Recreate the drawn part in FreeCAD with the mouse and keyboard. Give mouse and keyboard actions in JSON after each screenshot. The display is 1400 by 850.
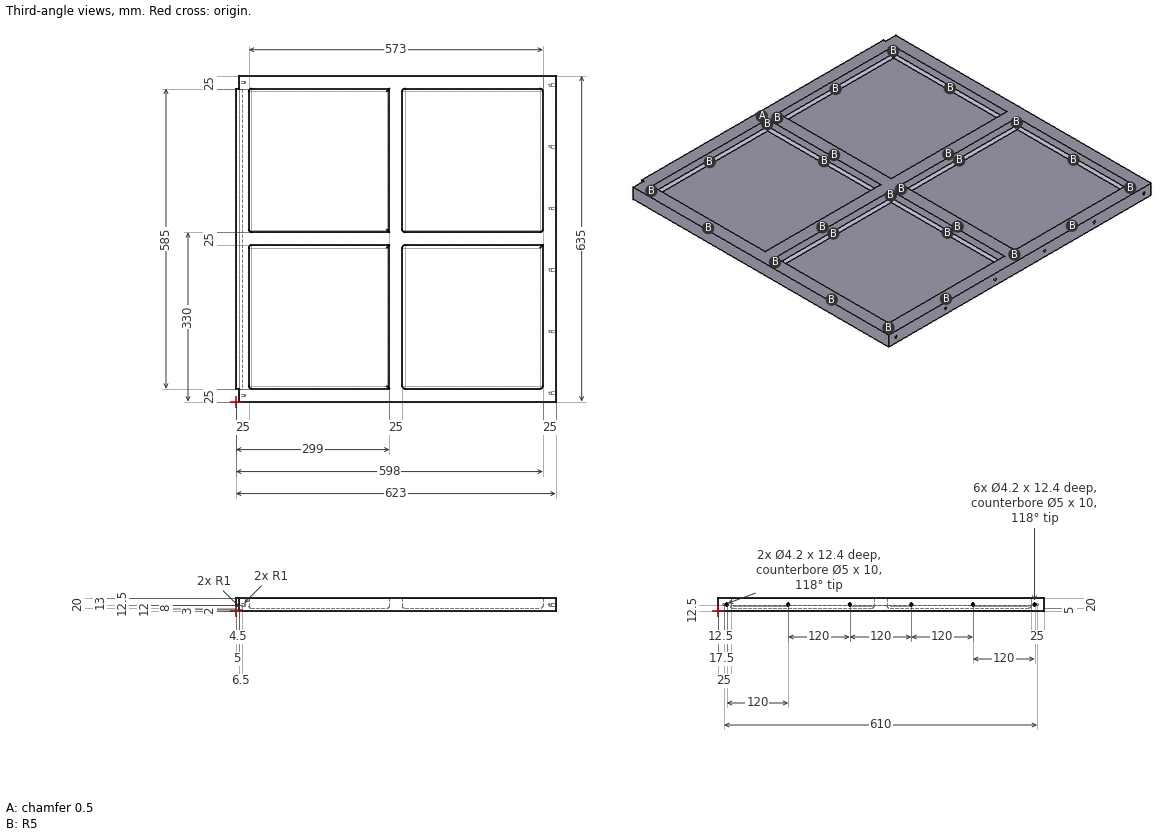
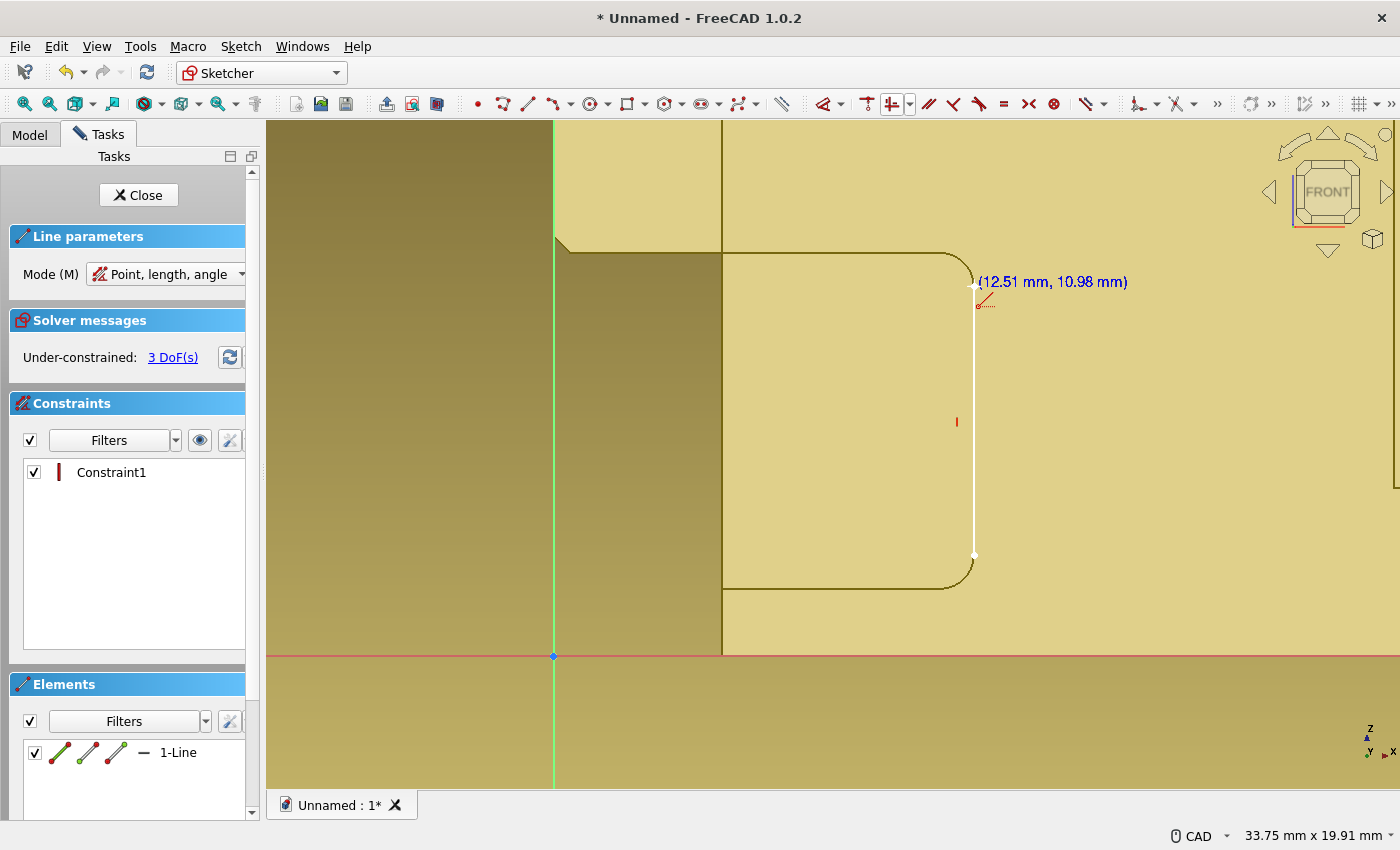
{"action": "key", "text": "g m"}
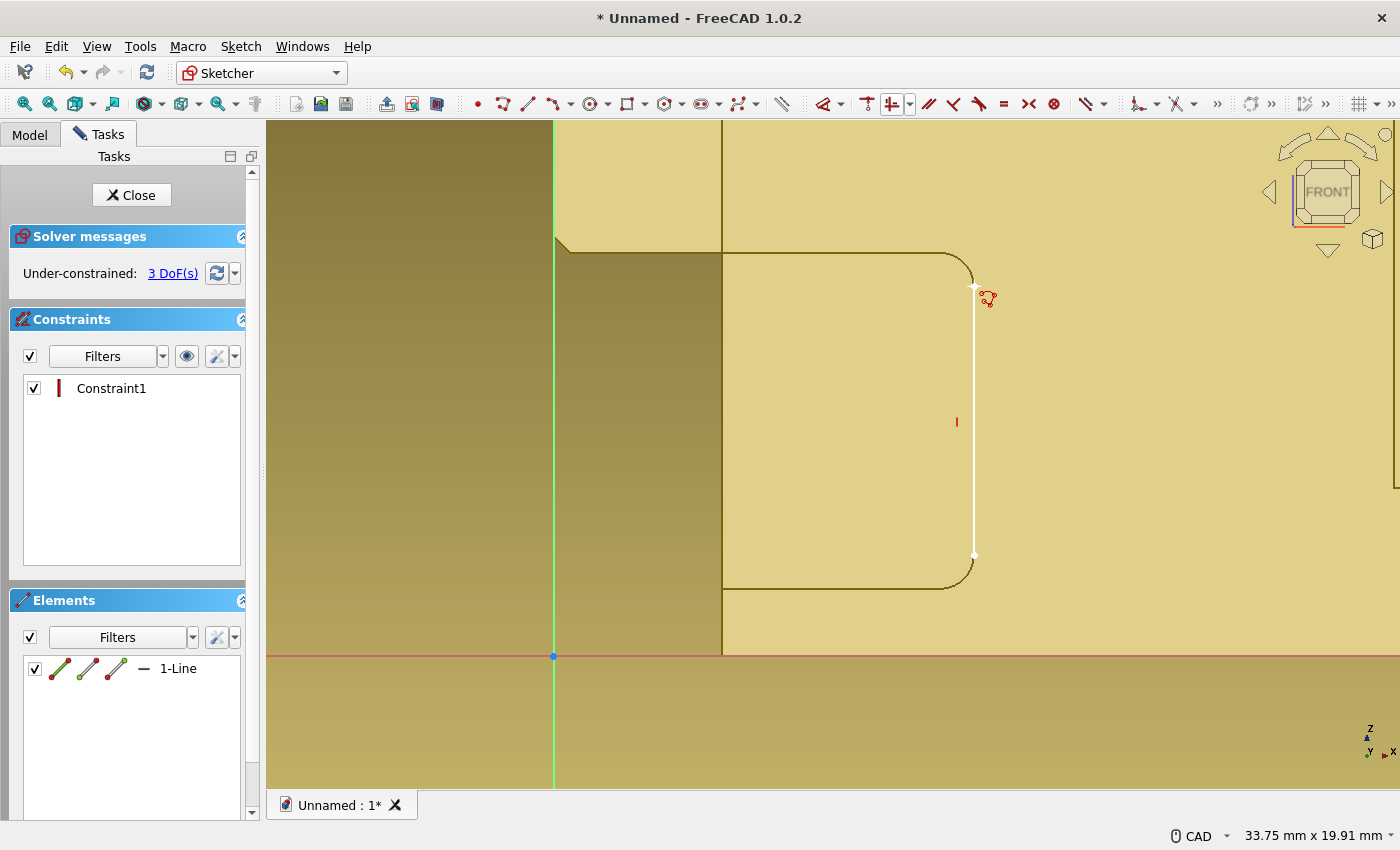
{"action": "left_click", "coordinate": [940, 253]}
{"action": "left_click", "coordinate": [722, 253]}
{"action": "left_click", "coordinate": [722, 589]}
{"action": "left_click", "coordinate": [940, 589]}
{"action": "right_click", "coordinate": [940, 589]}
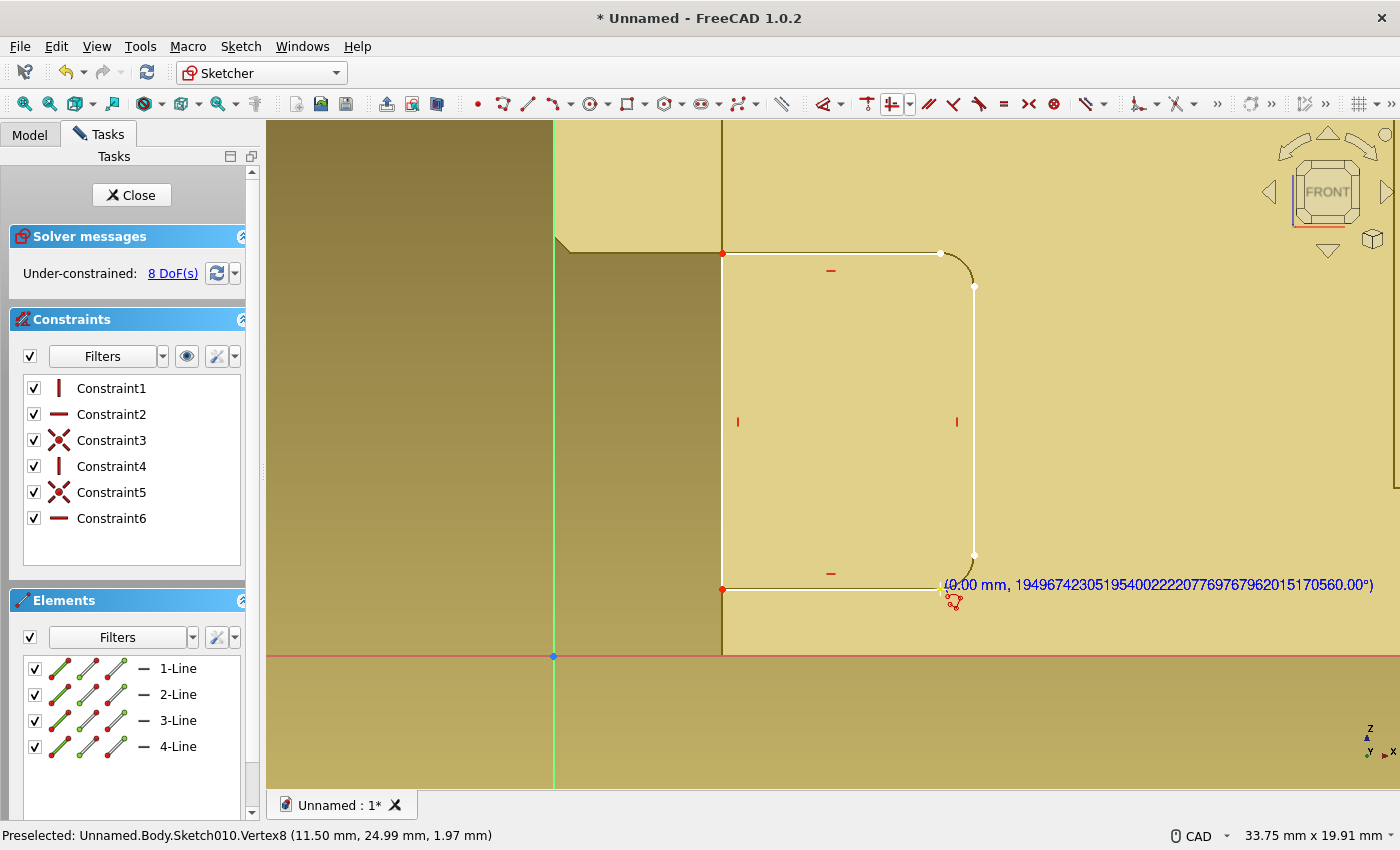
{"action": "key", "text": "g 3 a"}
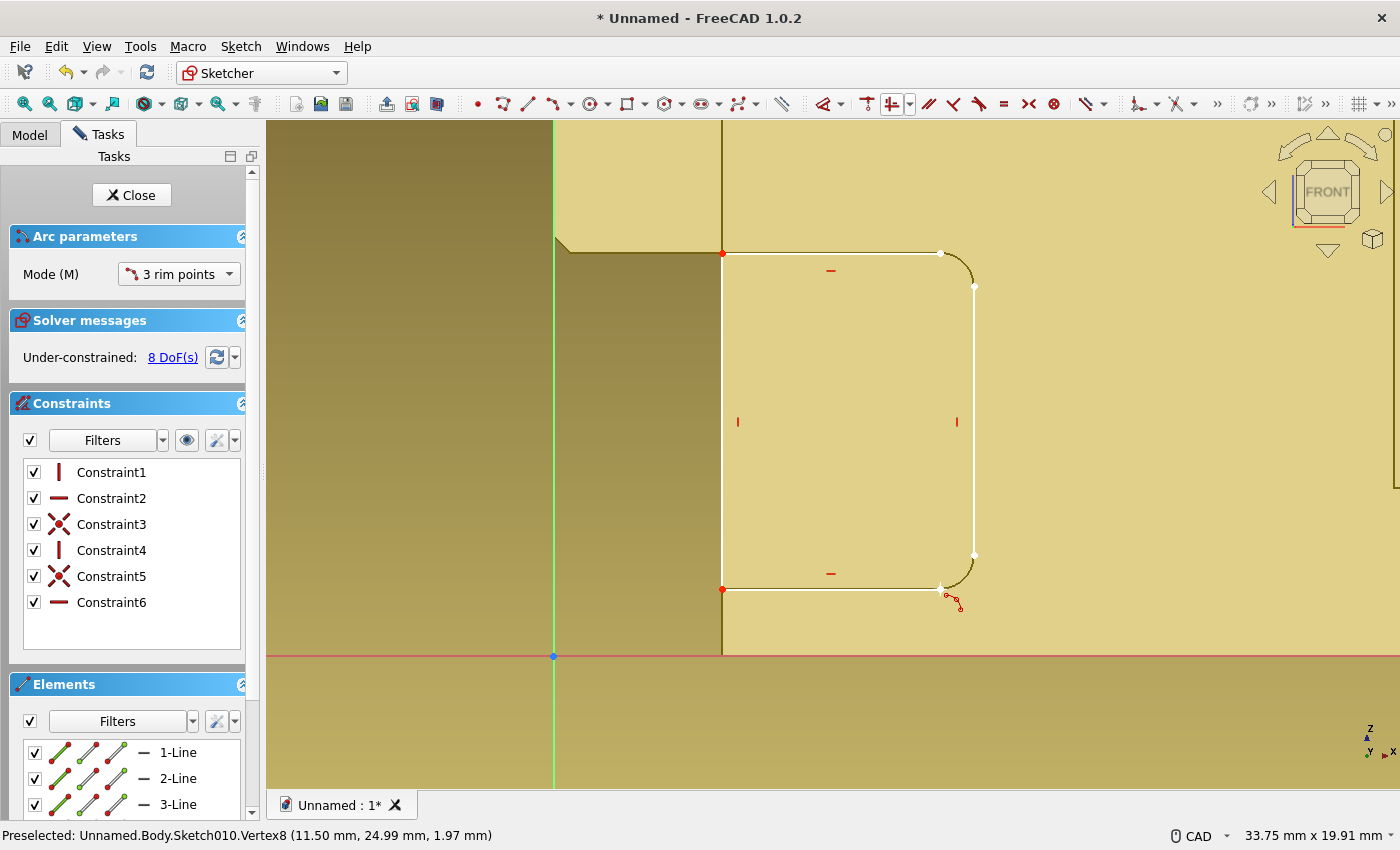
{"action": "left_click", "coordinate": [974, 287]}
{"action": "left_click", "coordinate": [940, 254]}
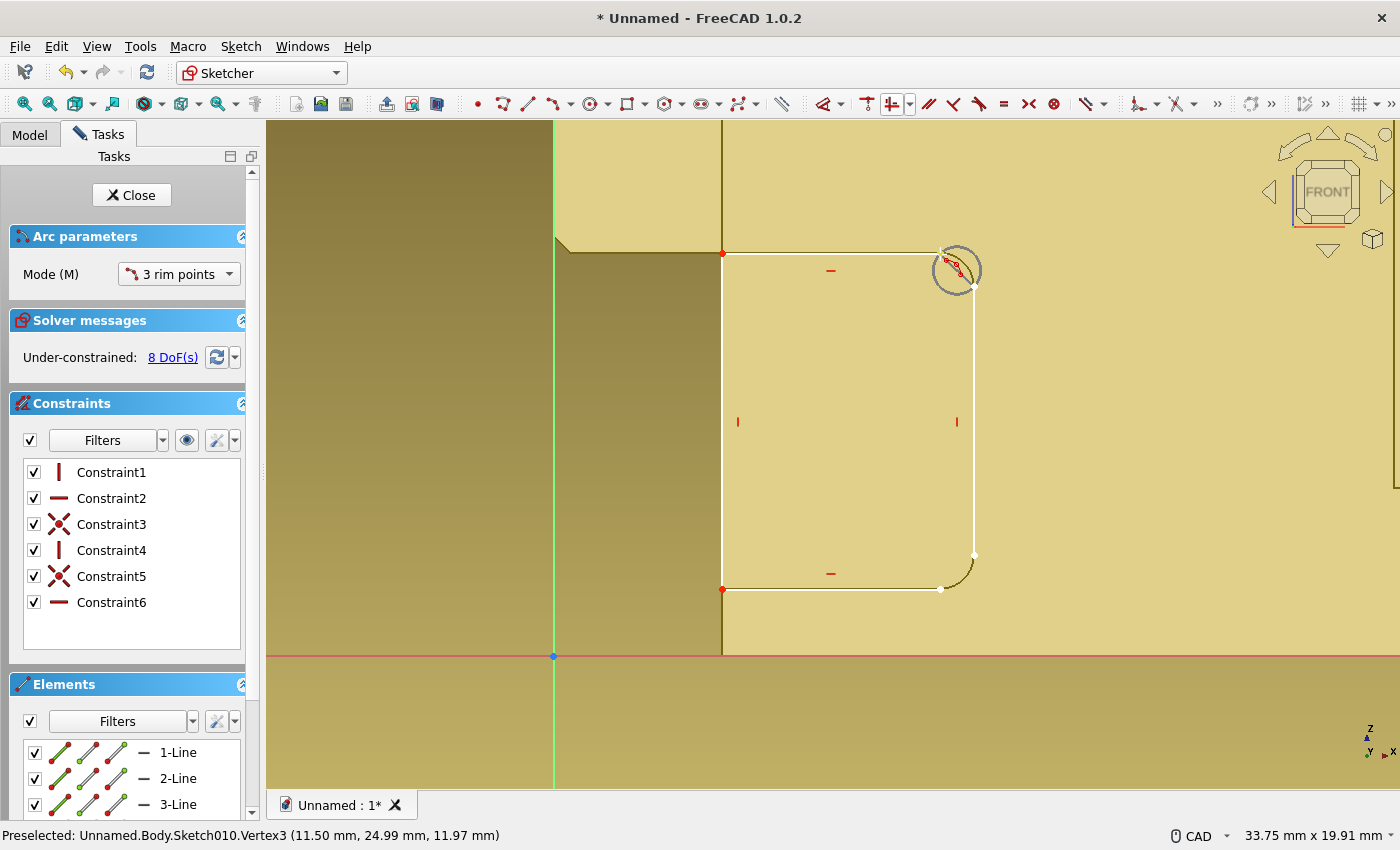
{"action": "scroll", "coordinate": [964, 263], "scroll_direction": "up", "scroll_amount": 3}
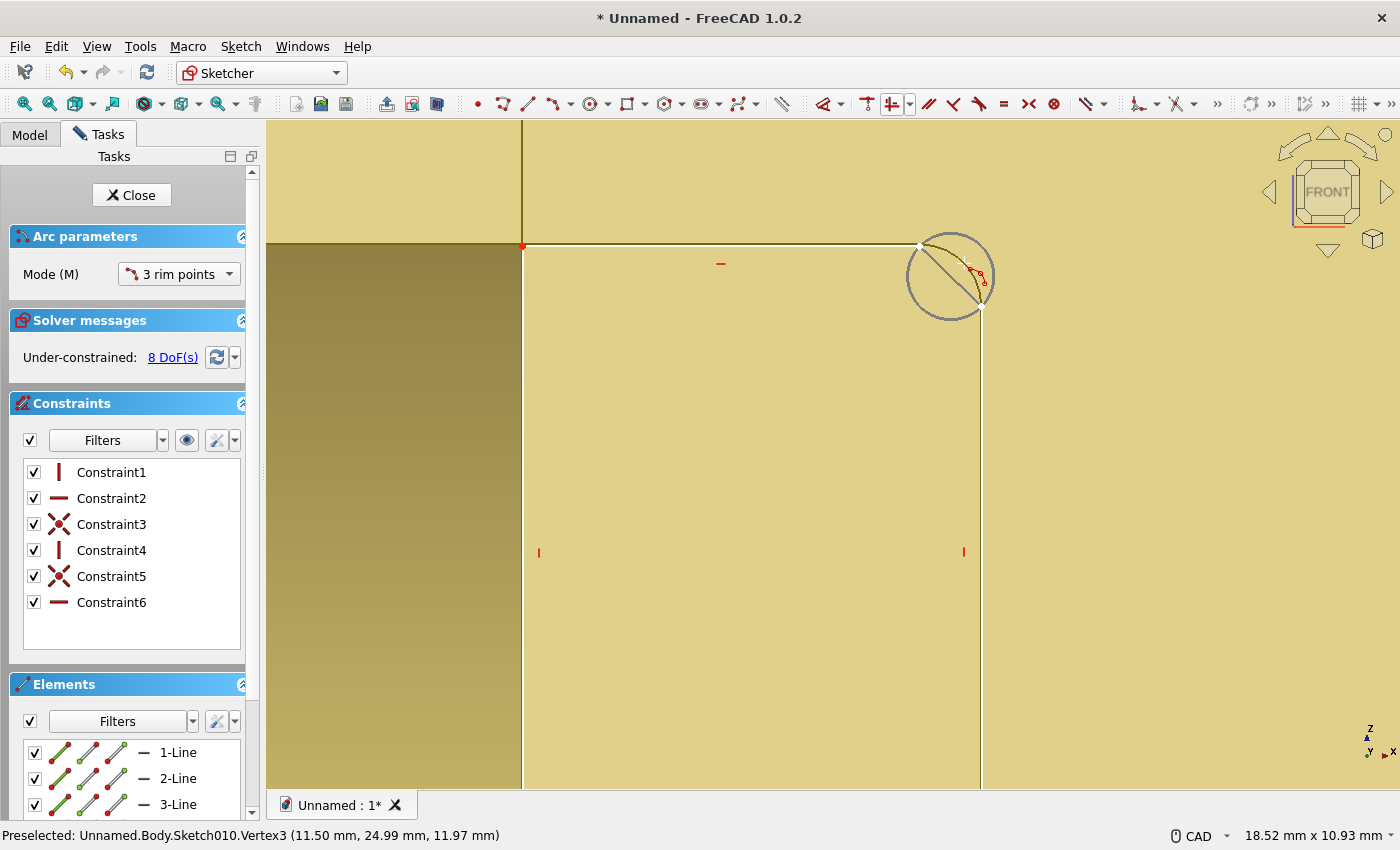
{"action": "left_click", "coordinate": [963, 262]}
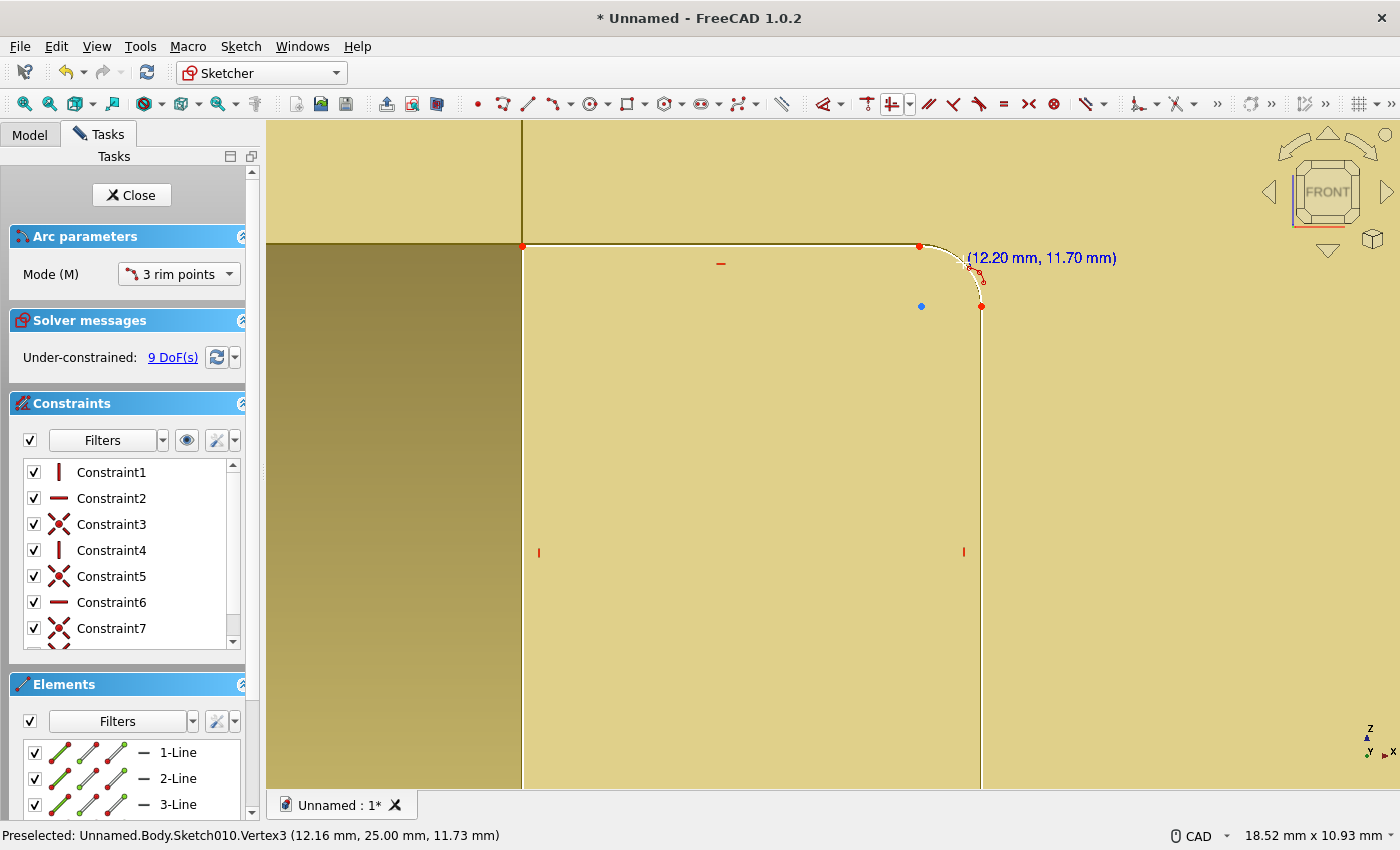
{"action": "scroll", "coordinate": [966, 263], "scroll_direction": "down", "scroll_amount": 3}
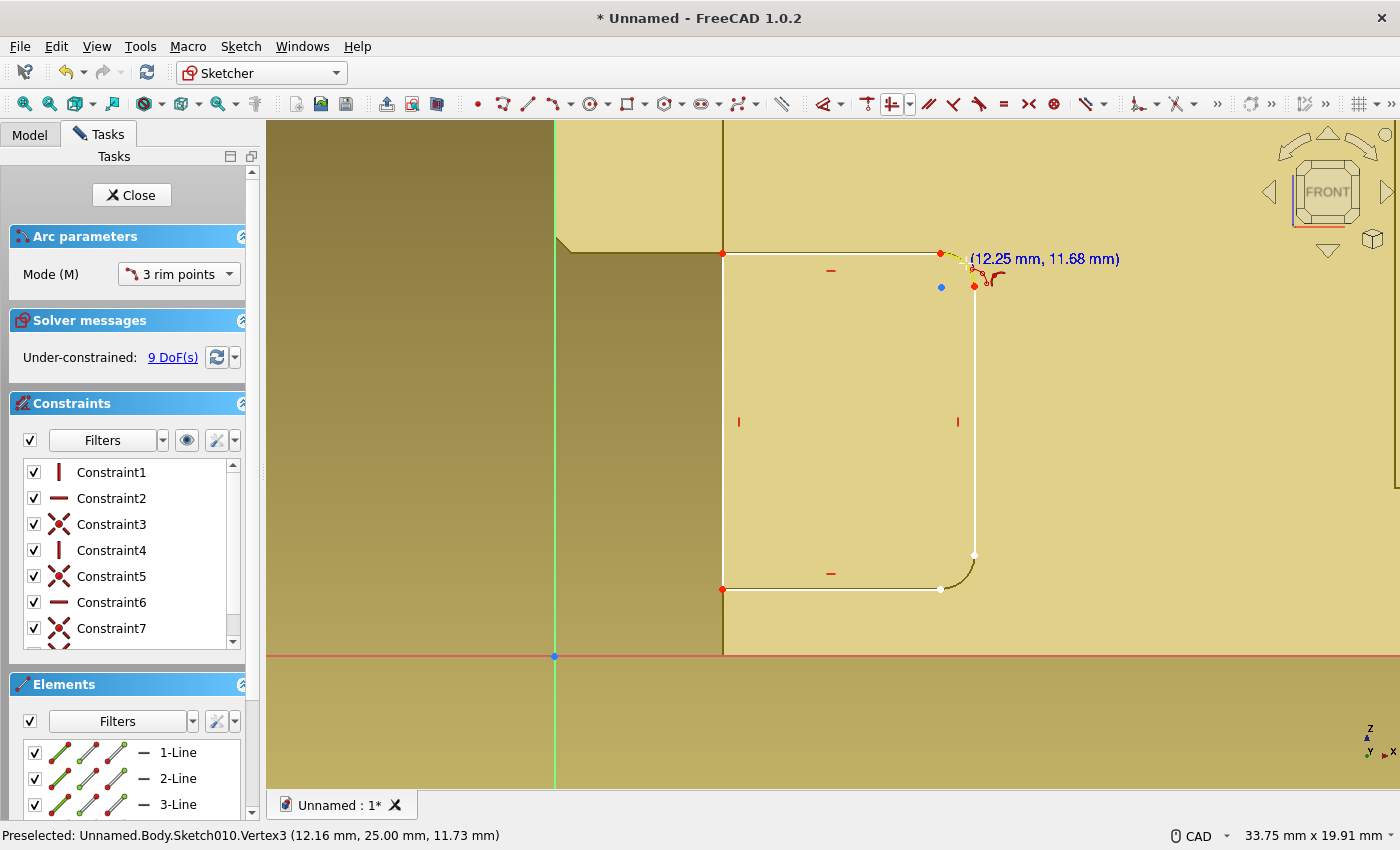
{"action": "left_click", "coordinate": [941, 590]}
{"action": "left_click", "coordinate": [975, 556]}